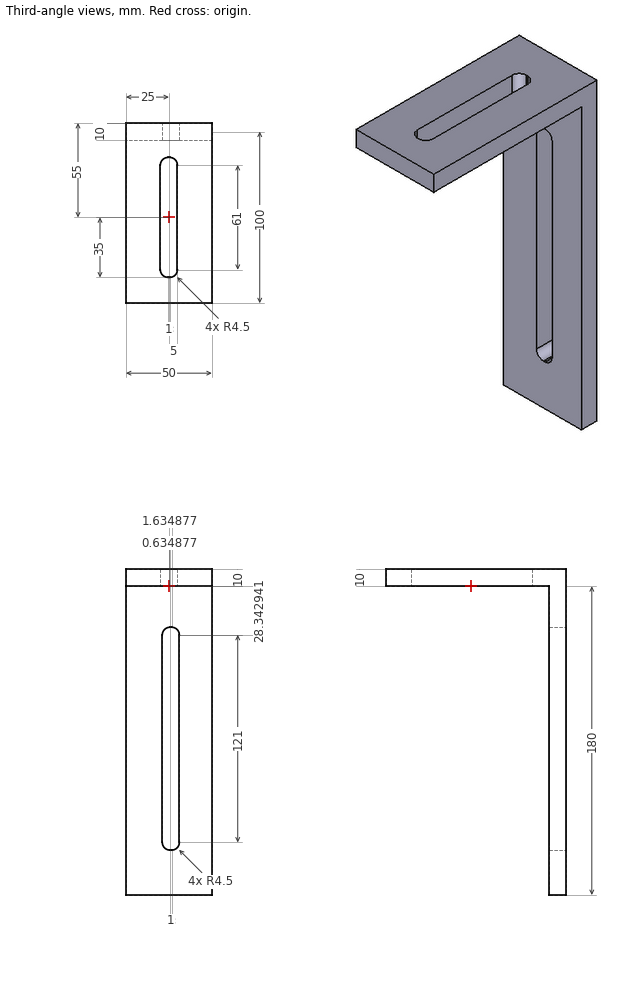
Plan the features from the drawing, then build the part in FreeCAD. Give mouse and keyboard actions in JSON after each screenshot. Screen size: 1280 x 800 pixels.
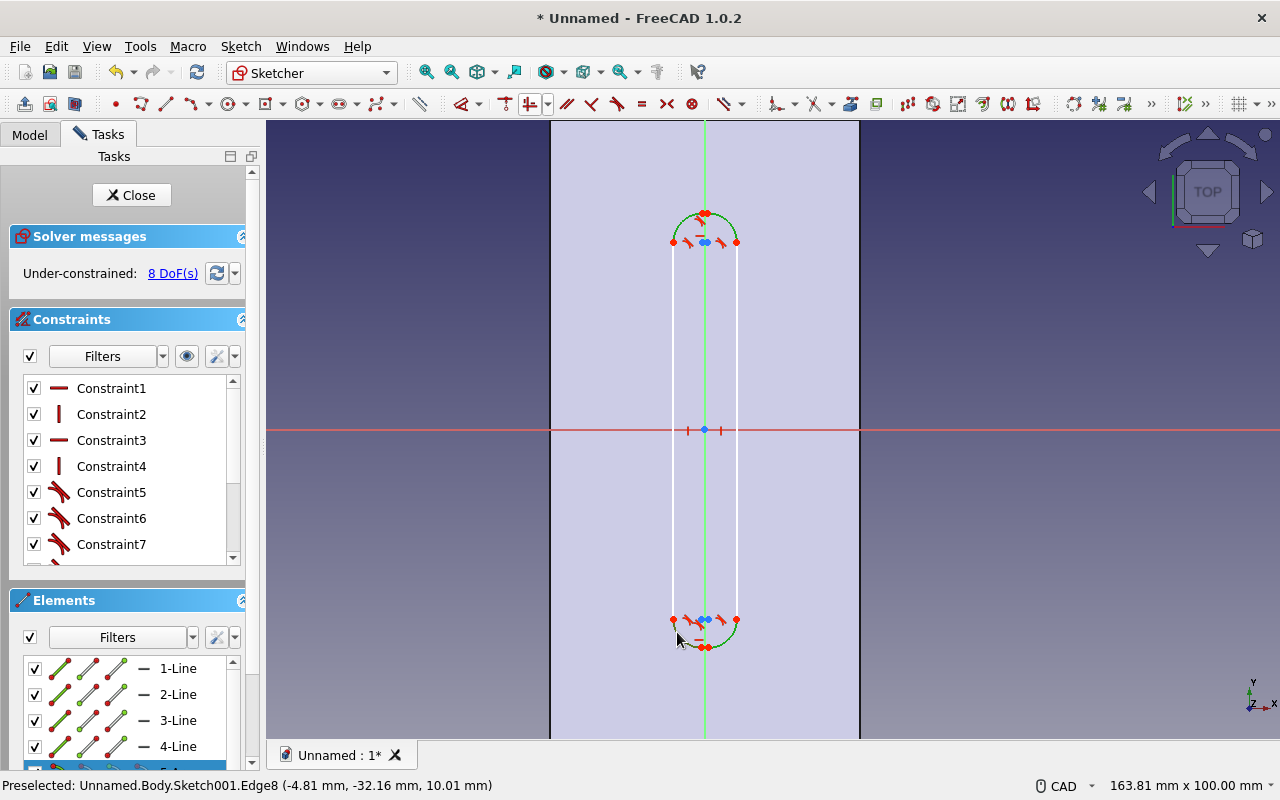
{"action": "left_click", "coordinate": [642, 104]}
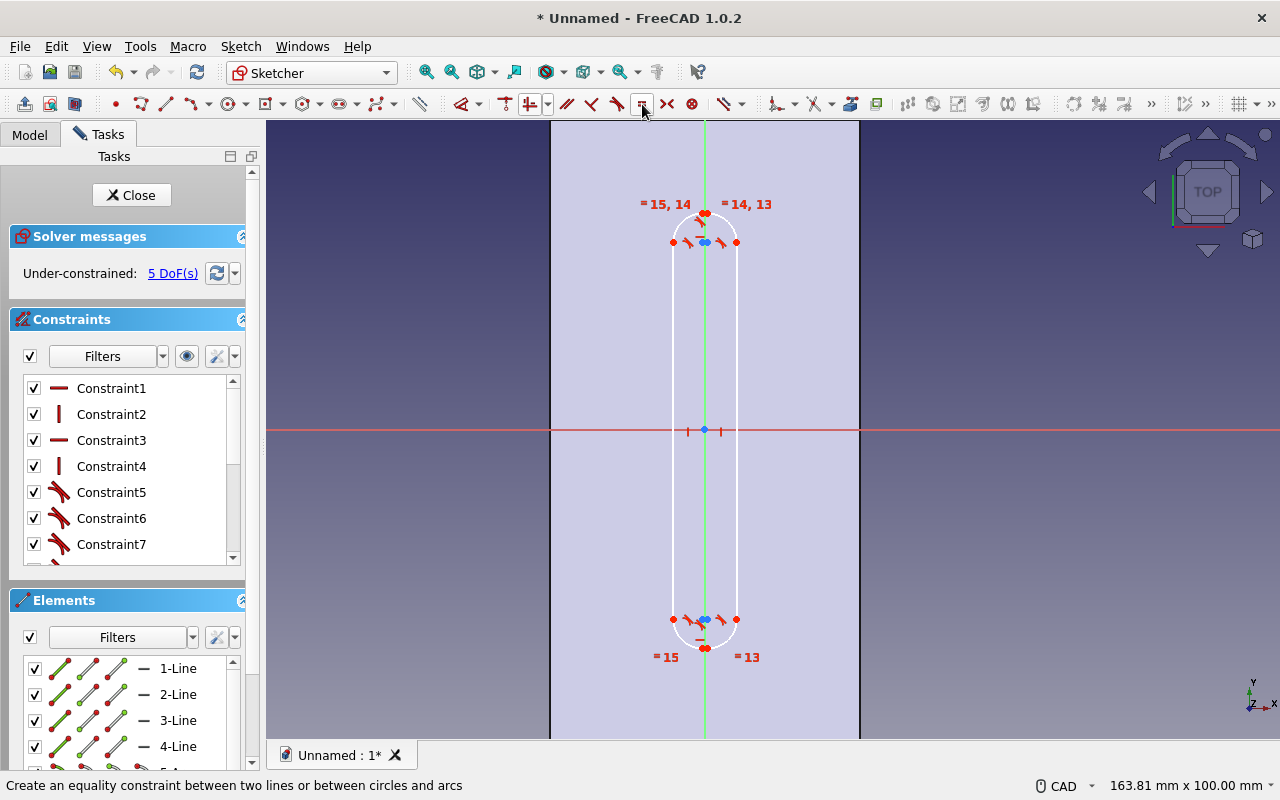
{"action": "left_click", "coordinate": [460, 104]}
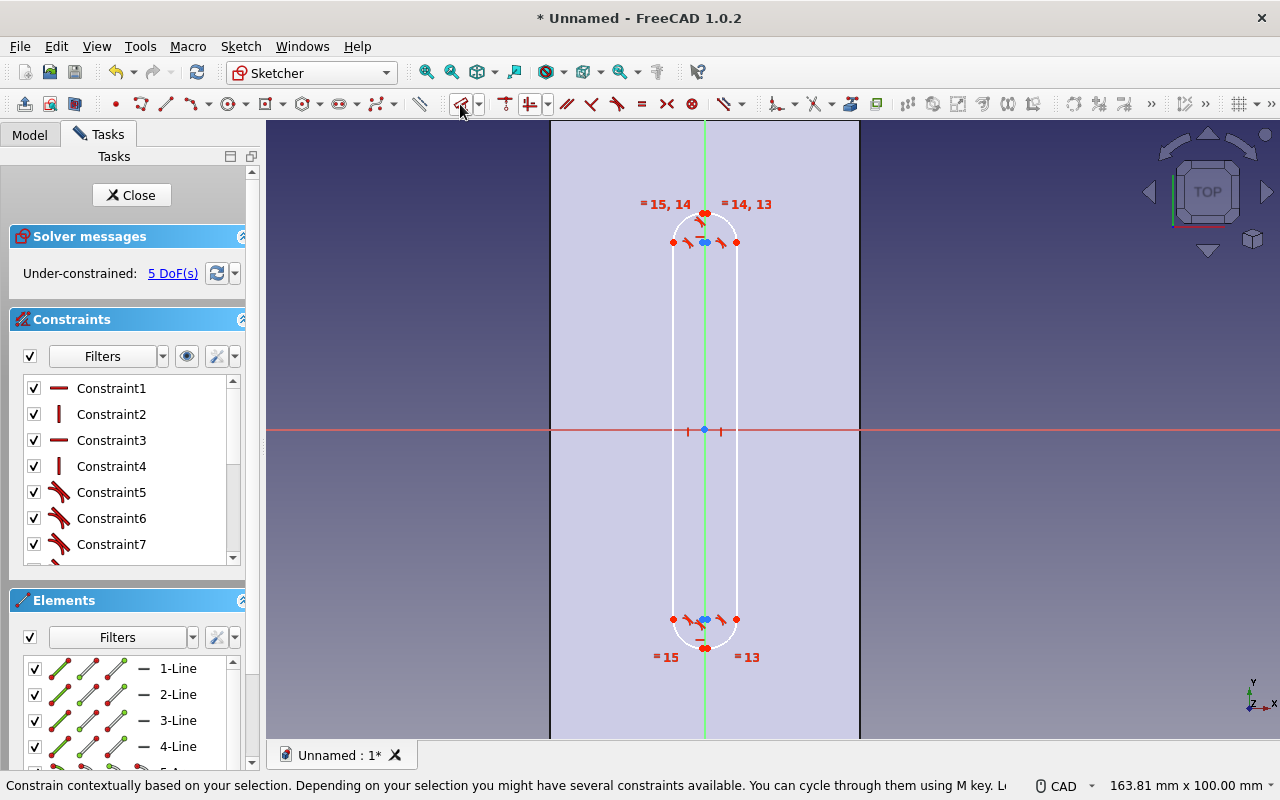
{"action": "scroll", "coordinate": [721, 645], "scroll_direction": "up", "scroll_amount": 2}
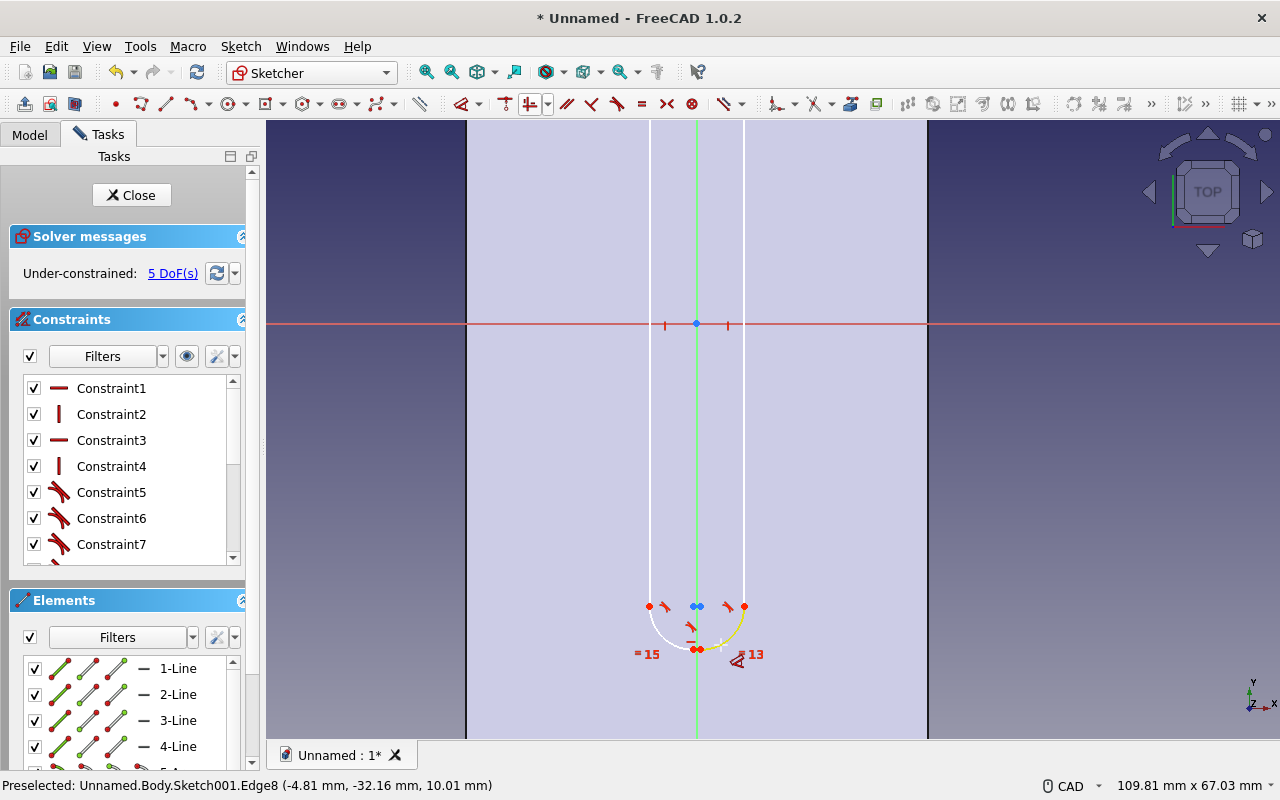
{"action": "left_click", "coordinate": [721, 645]}
{"action": "left_click", "coordinate": [736, 673]}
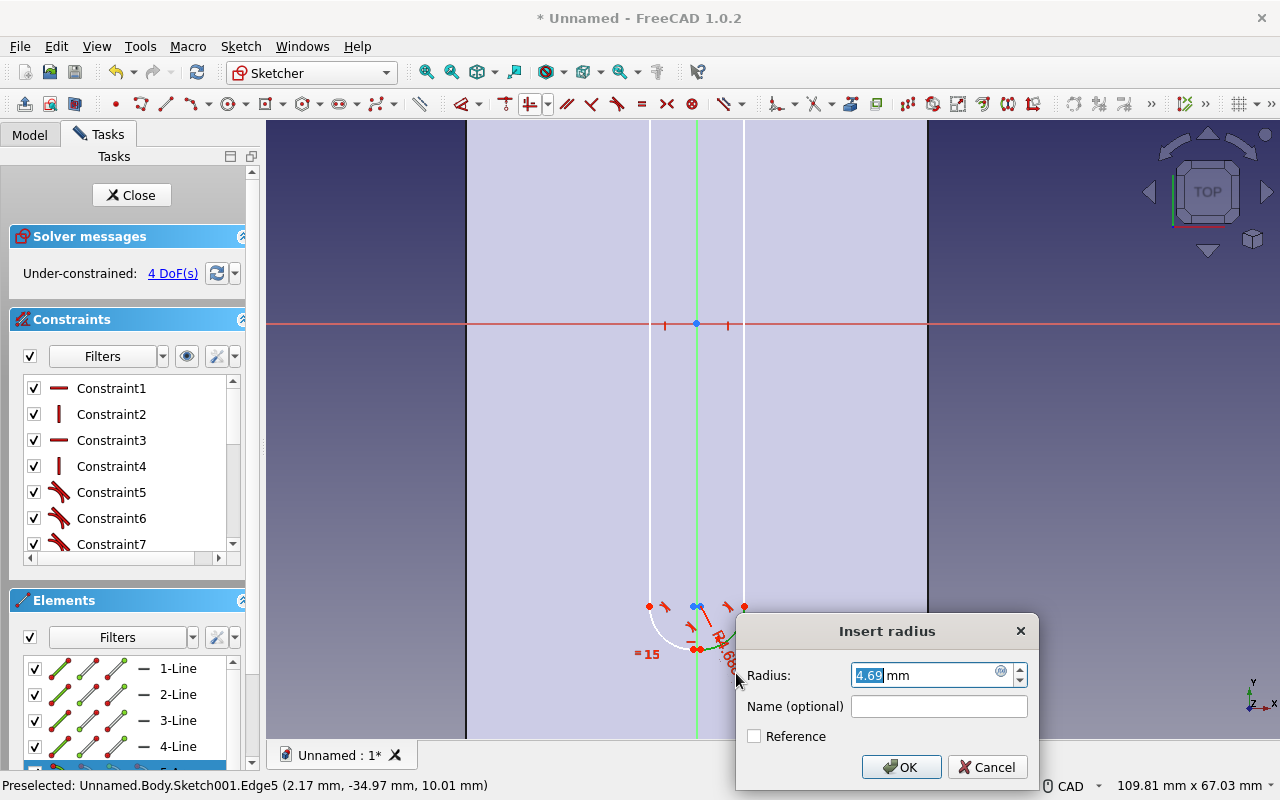
{"action": "type", "text": "4.5"}
{"action": "key", "text": "Return"}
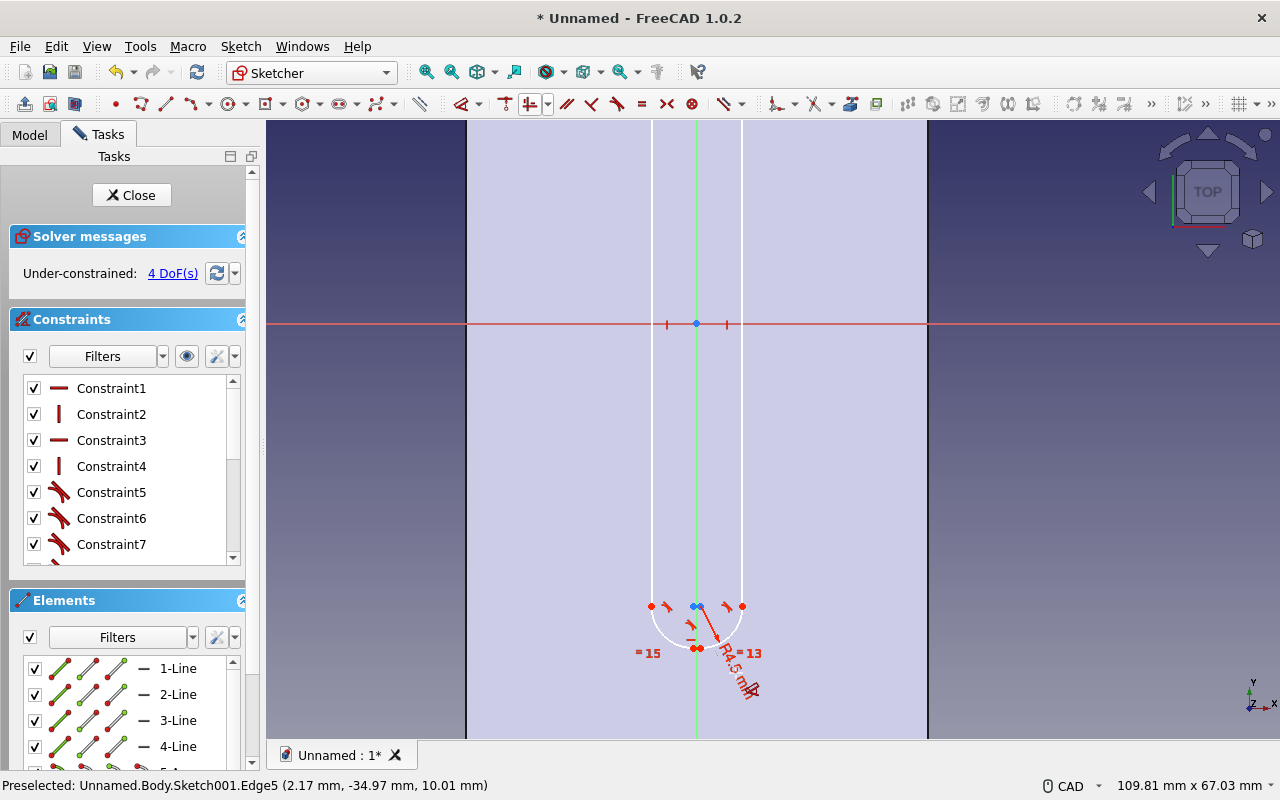
{"action": "scroll", "coordinate": [697, 648], "scroll_direction": "up", "scroll_amount": 8}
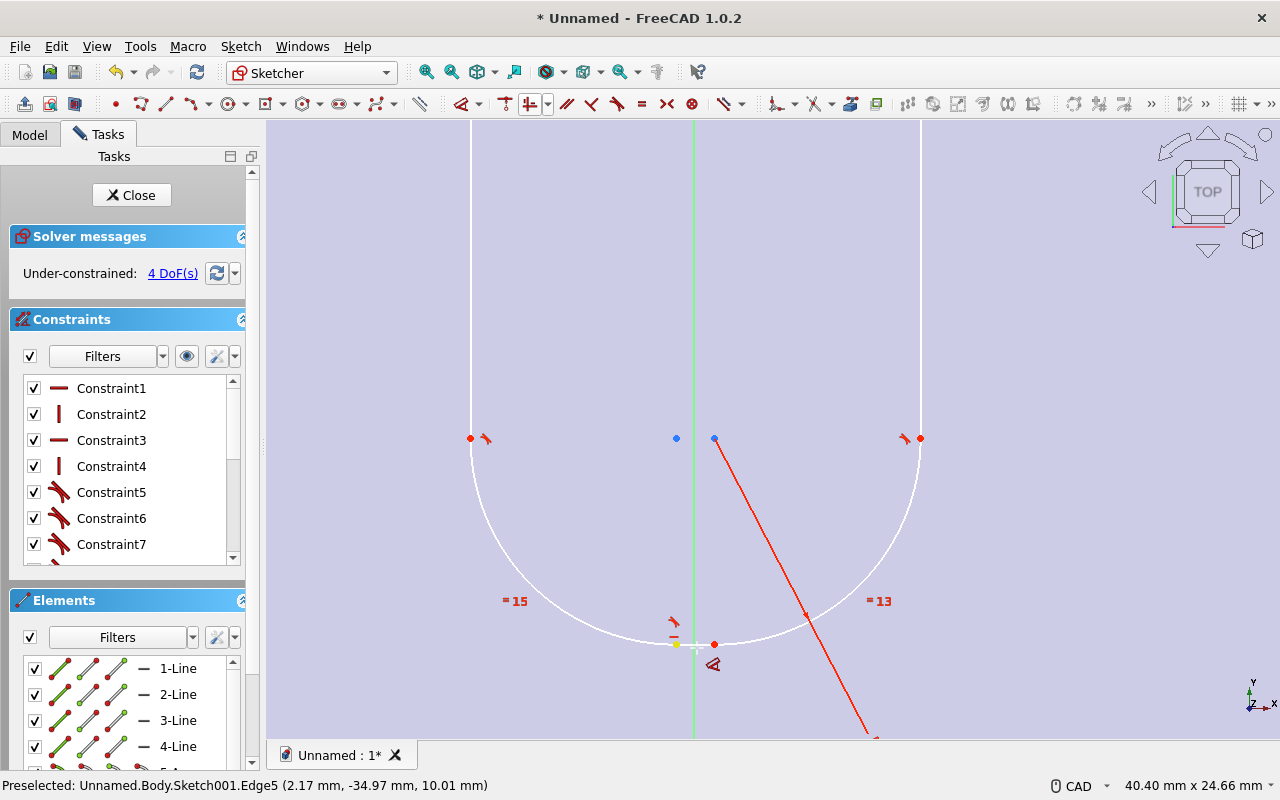
{"action": "left_click", "coordinate": [696, 645]}
{"action": "left_click", "coordinate": [709, 679]}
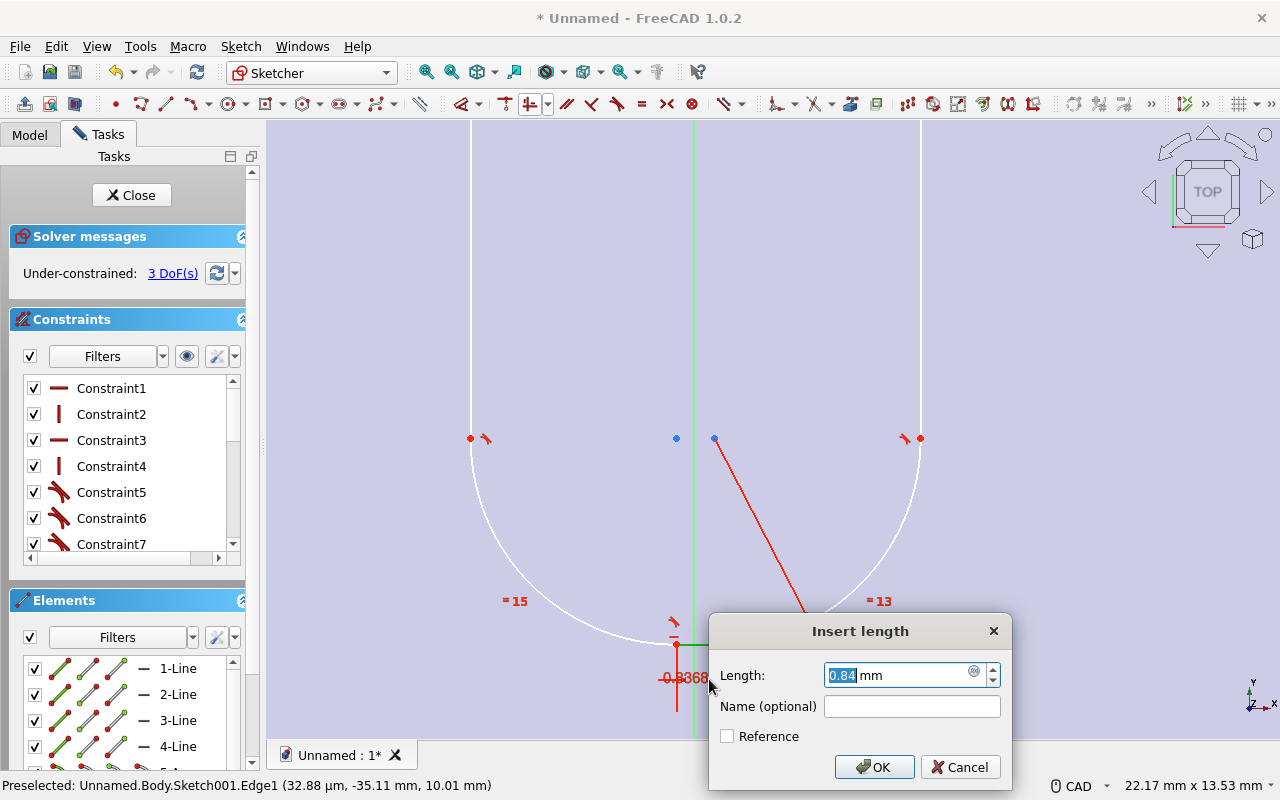
{"action": "type", "text": "1"}
{"action": "key", "text": "Return"}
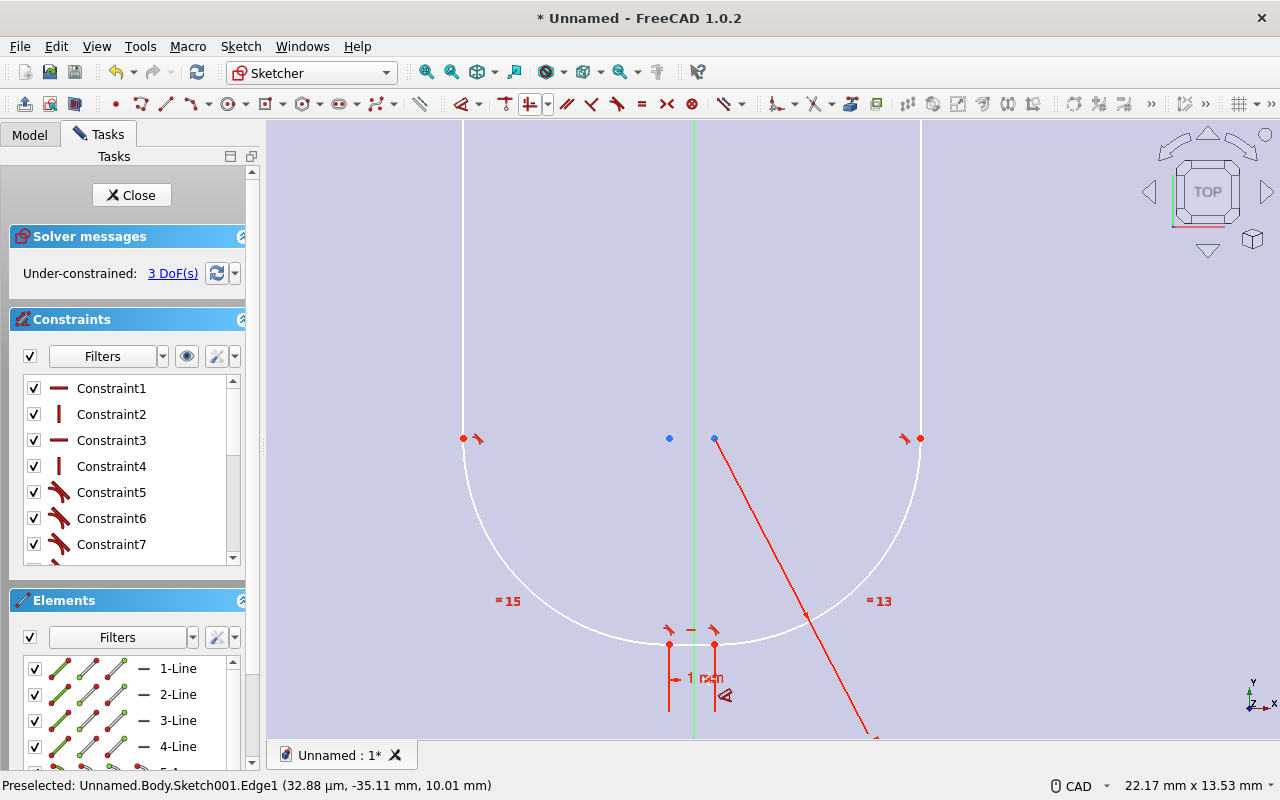
{"action": "scroll", "coordinate": [706, 647], "scroll_direction": "down", "scroll_amount": 10}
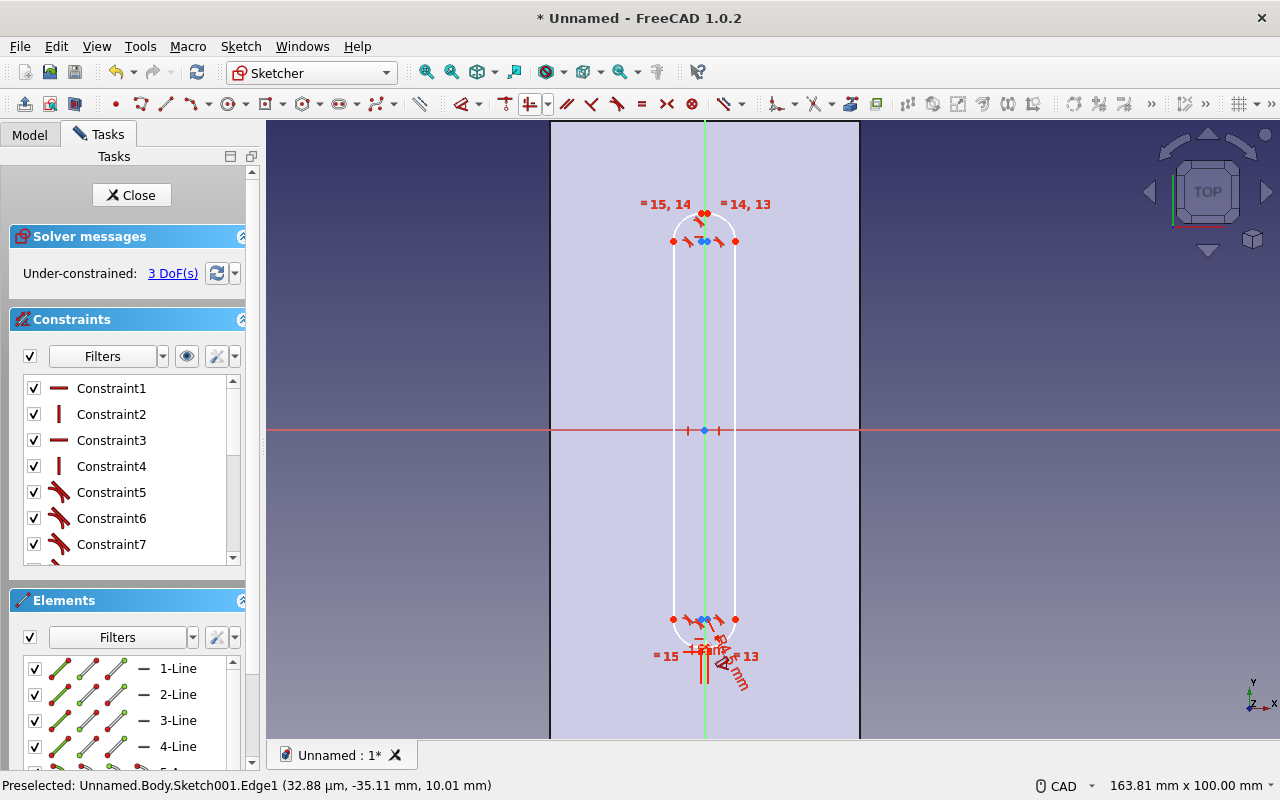
{"action": "left_click", "coordinate": [735, 506]}
{"action": "left_click", "coordinate": [769, 344]}